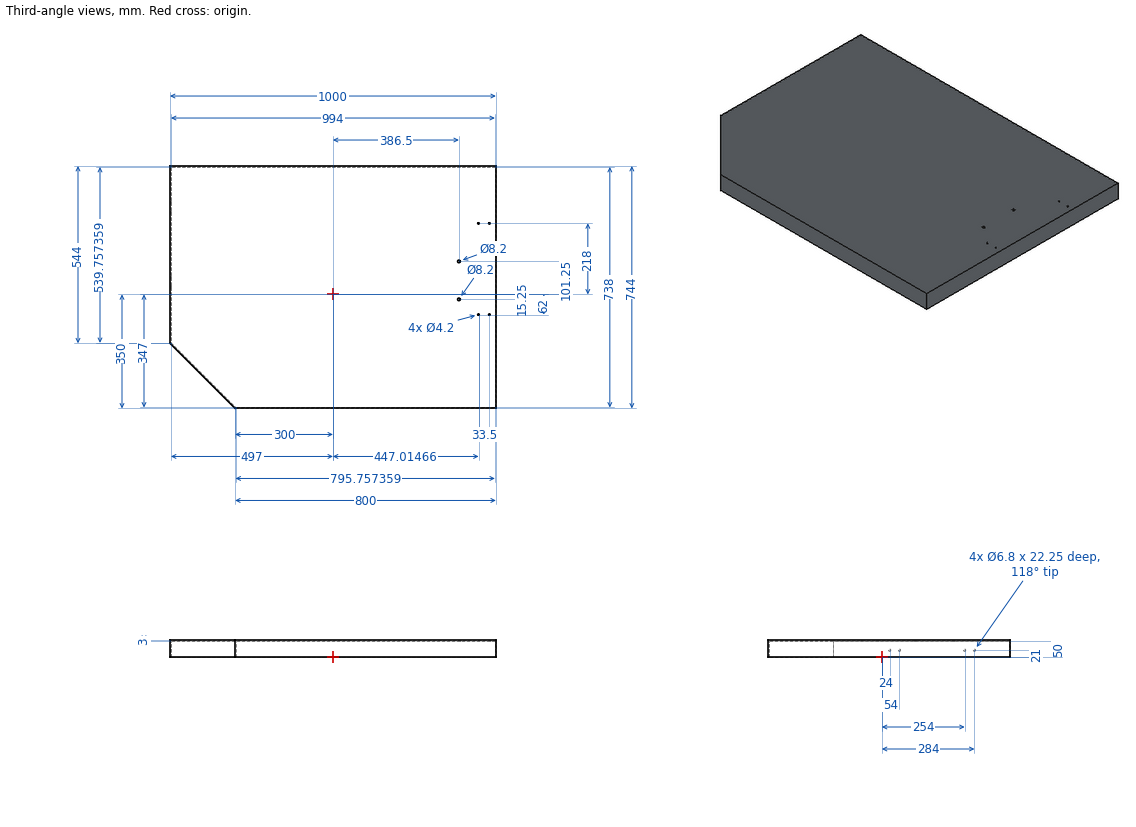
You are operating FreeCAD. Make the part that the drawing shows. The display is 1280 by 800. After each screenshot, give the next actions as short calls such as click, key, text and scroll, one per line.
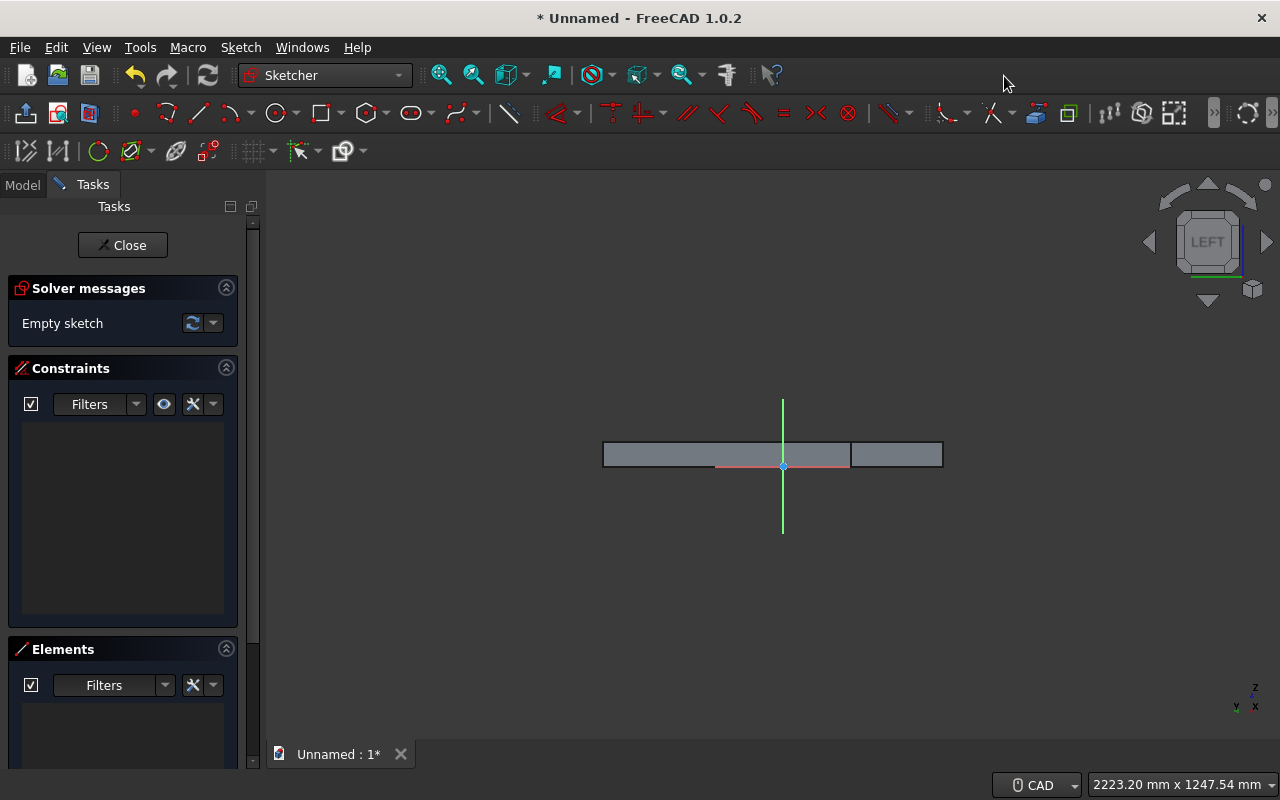
scroll(722, 463, up, 7)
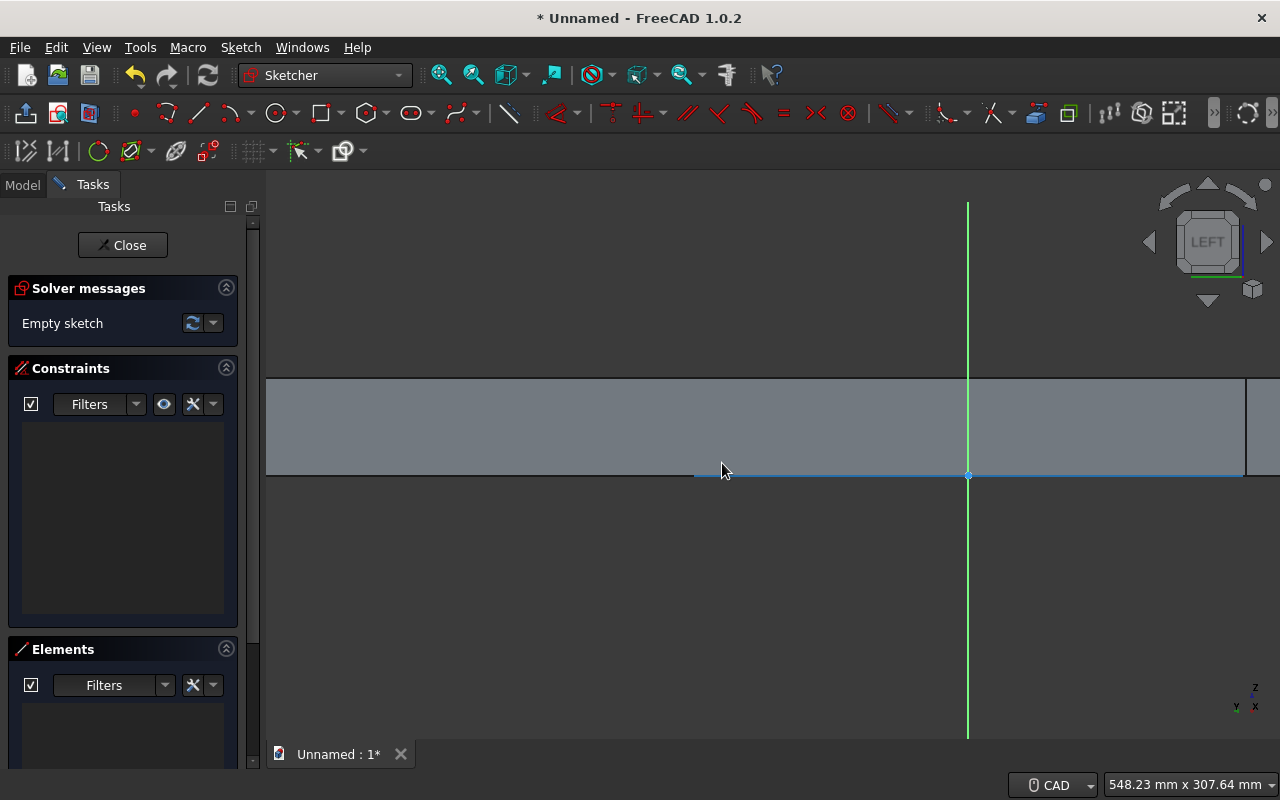
click(276, 114)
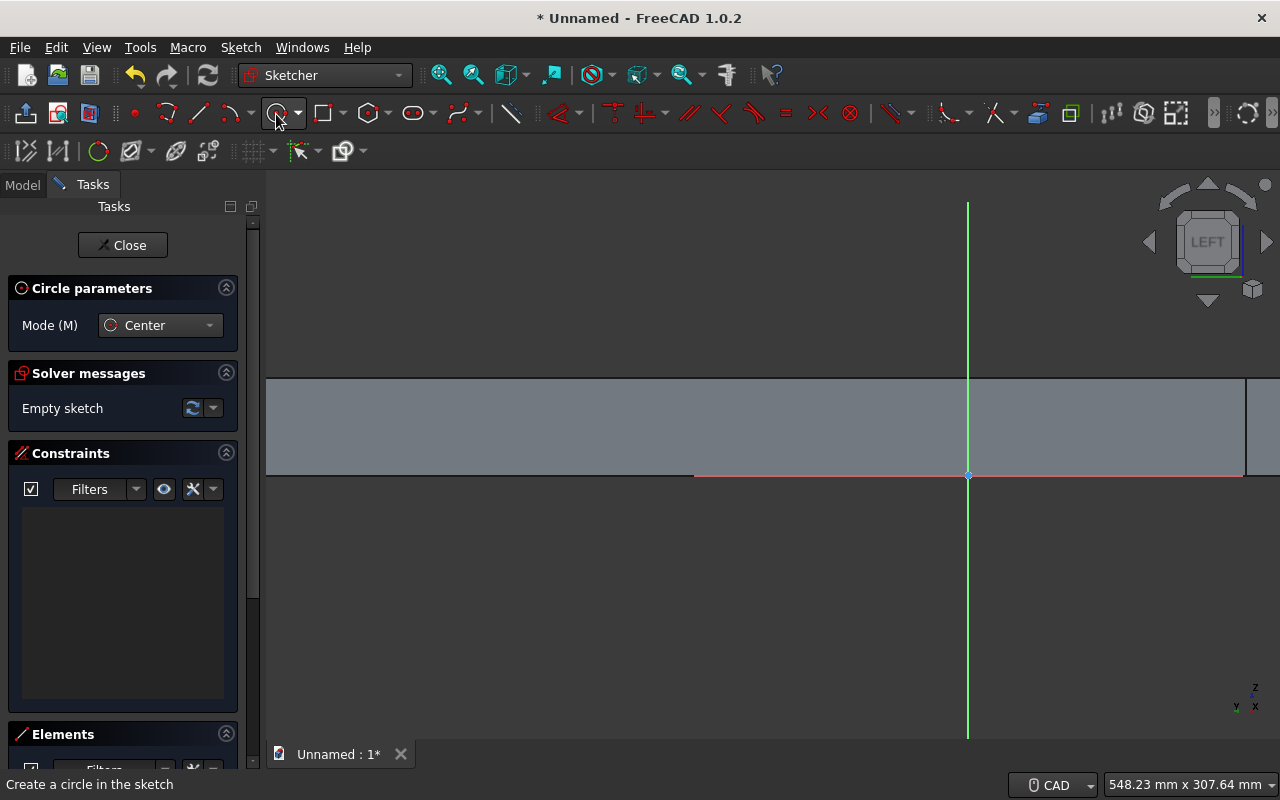
scroll(443, 437, up, 7)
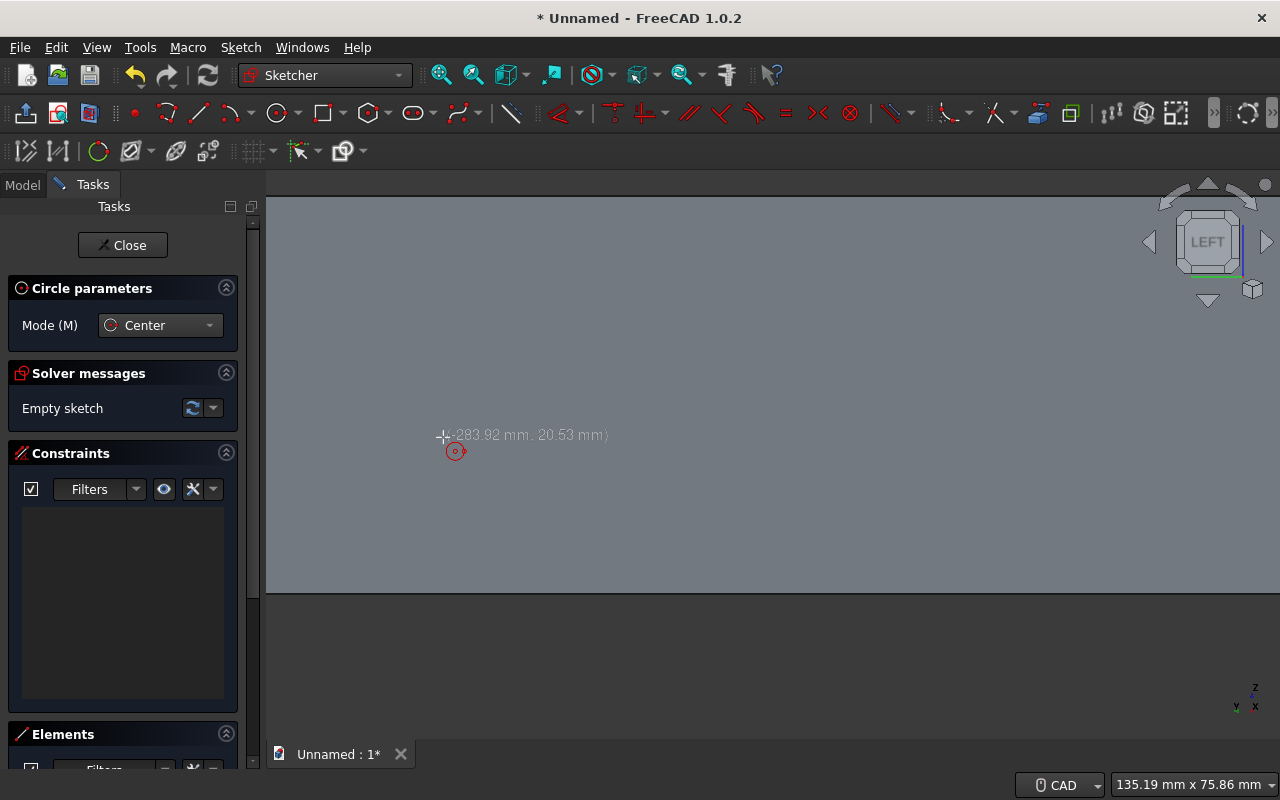
scroll(446, 439, down, 7)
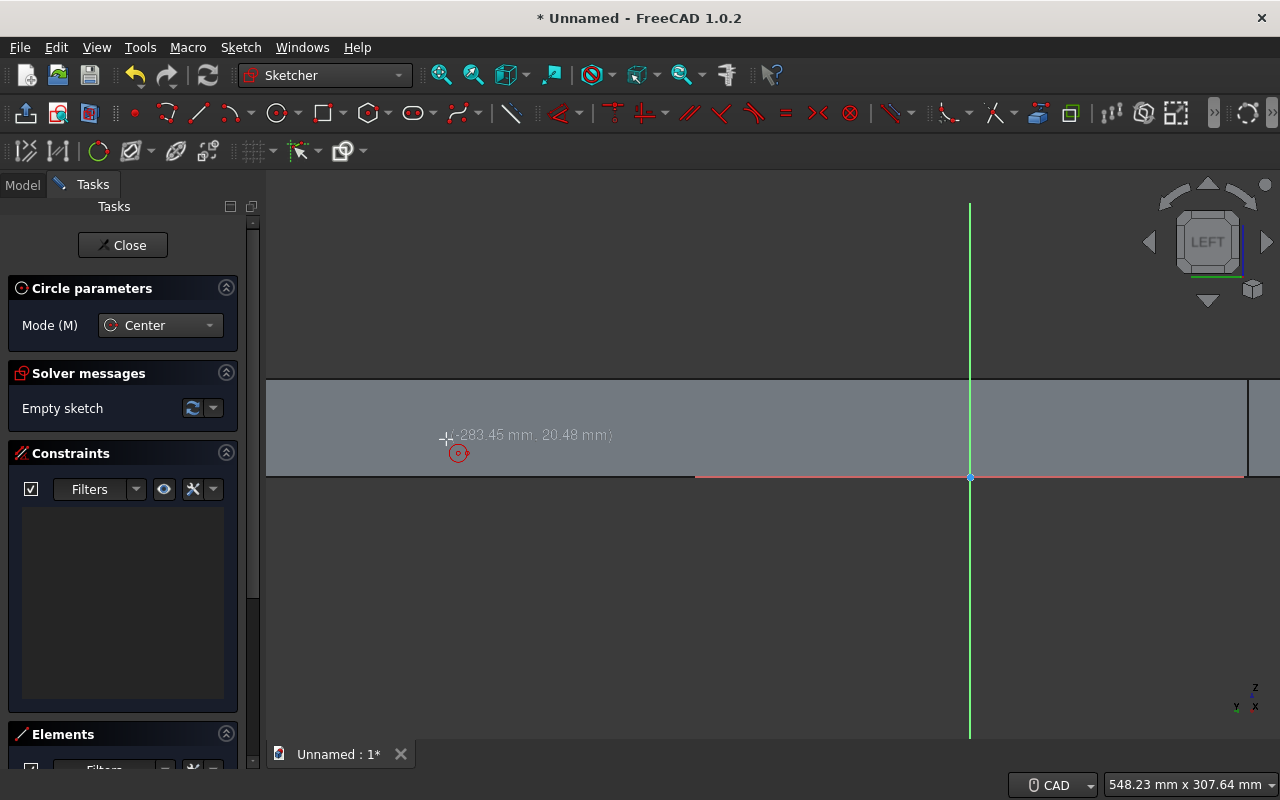
click(445, 439)
move(450, 434)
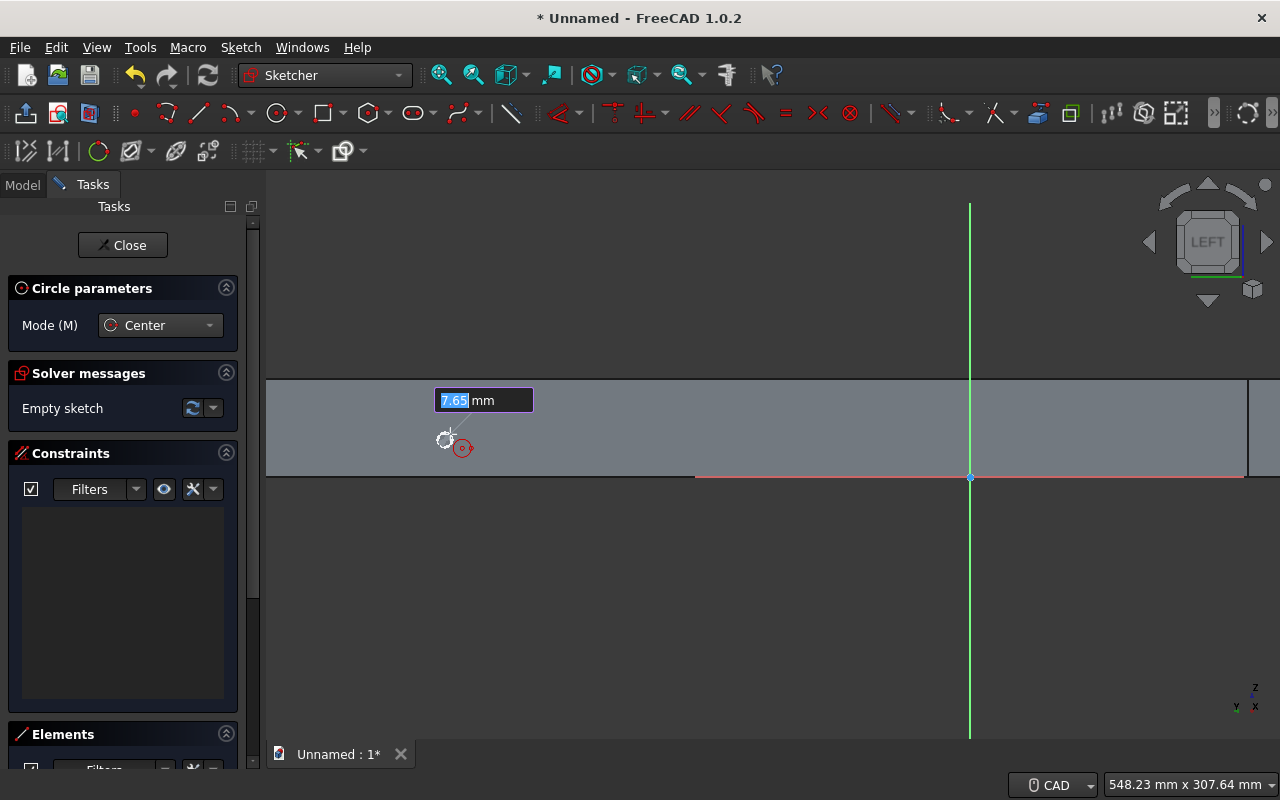
text(6.8)
key(Return)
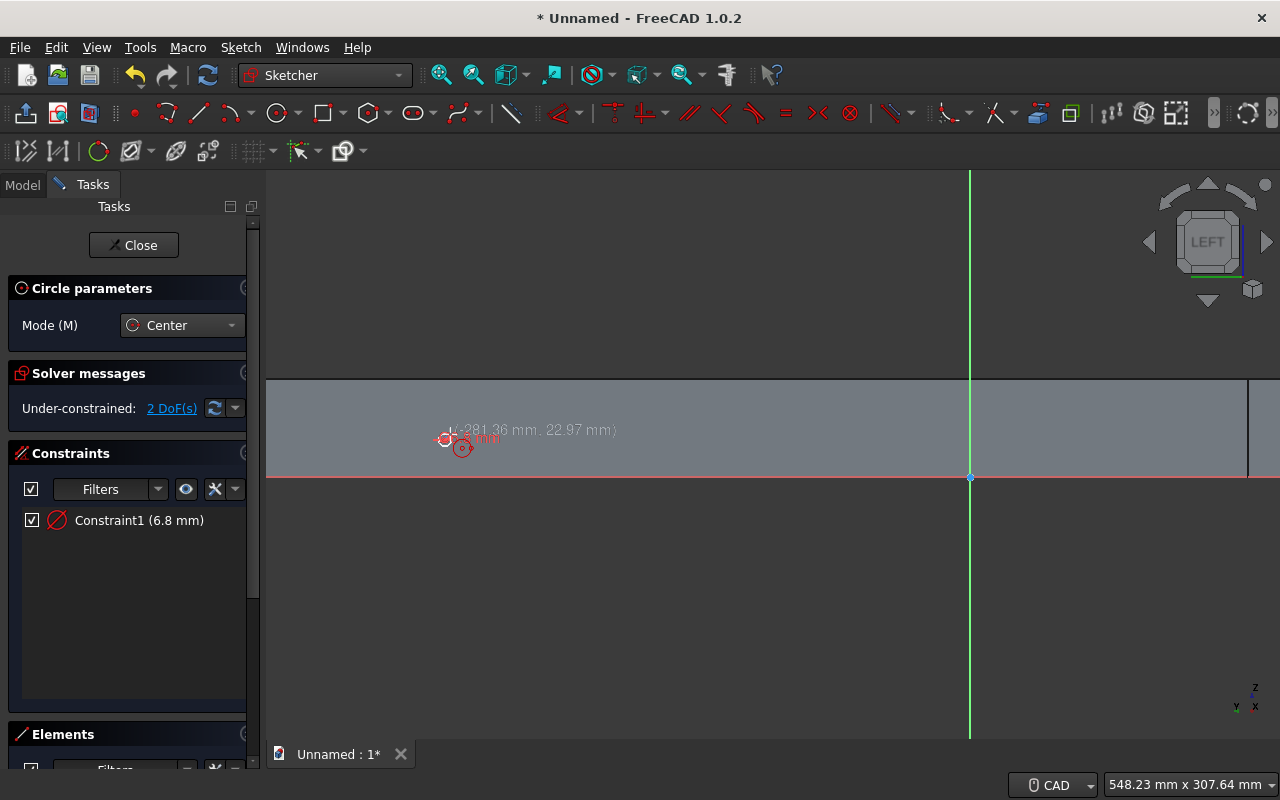
scroll(501, 439, up, 7)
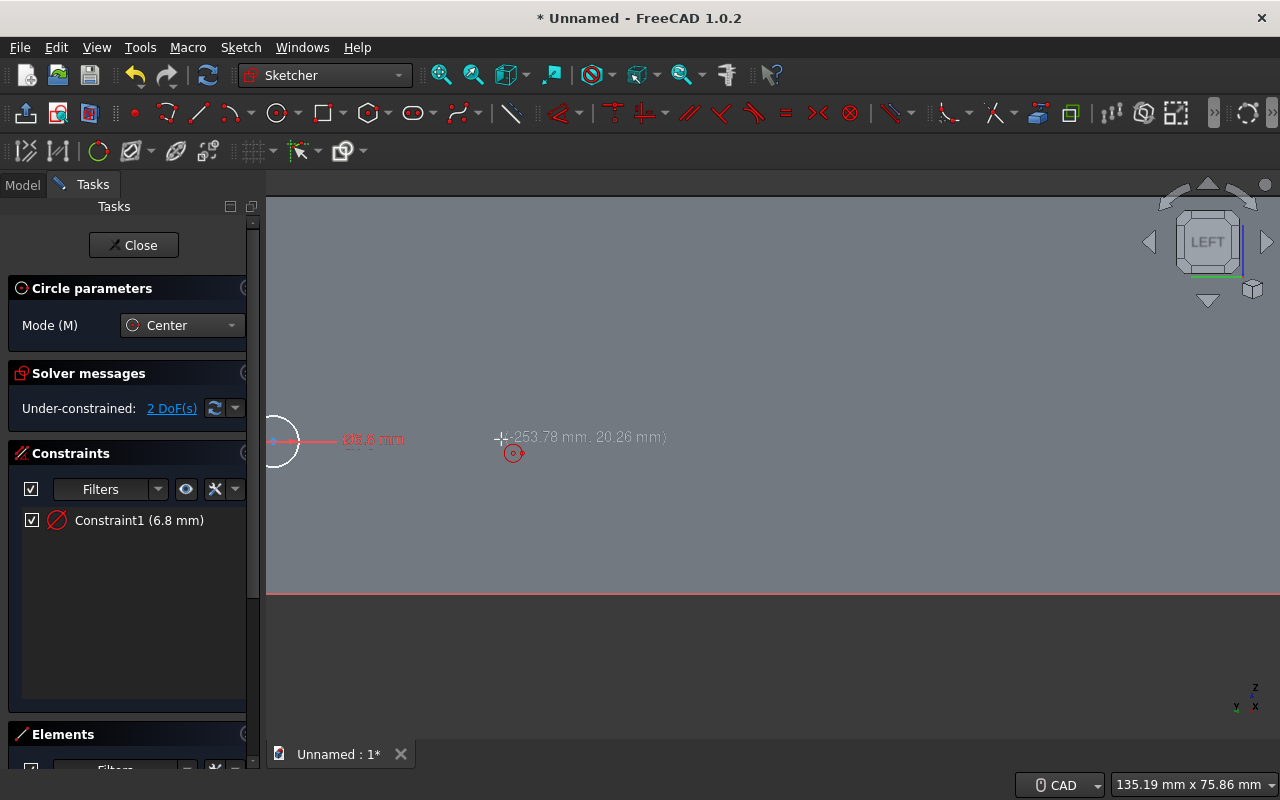
scroll(501, 439, down, 7)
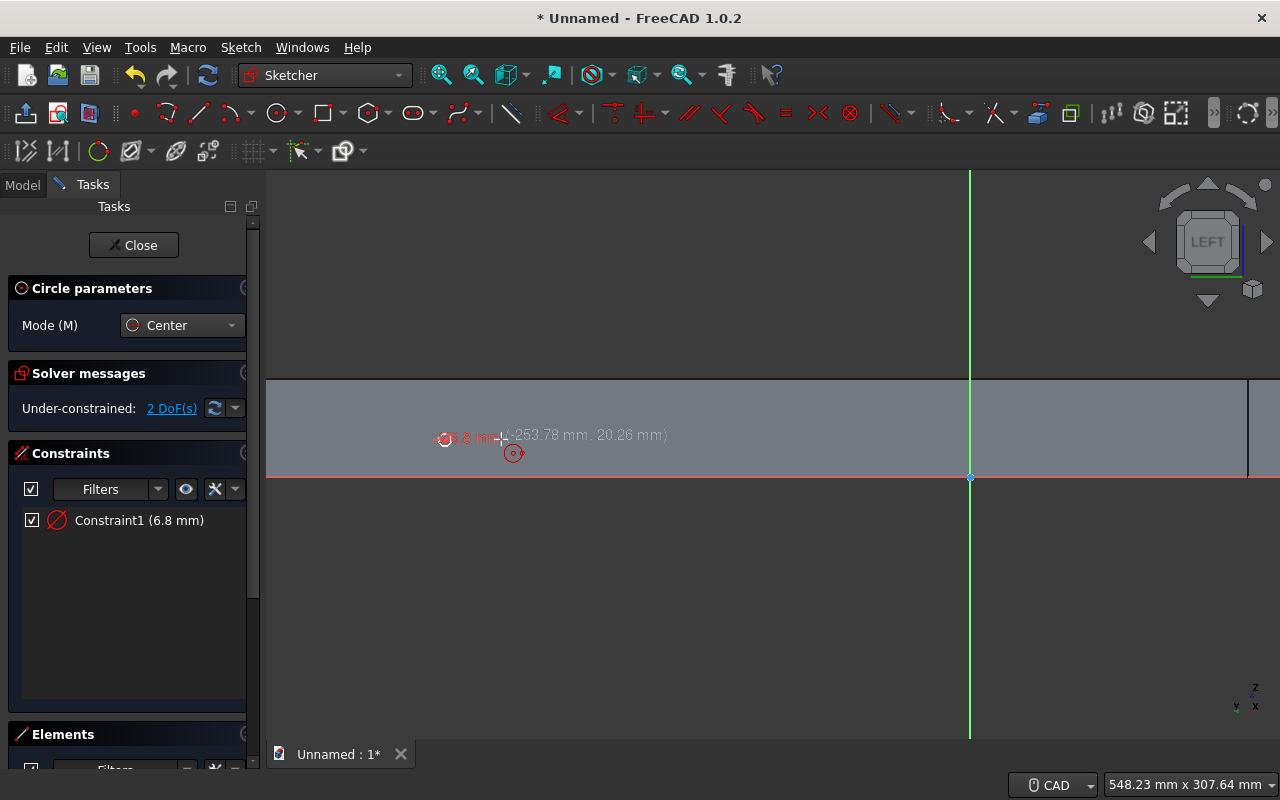
click(501, 439)
move(505, 434)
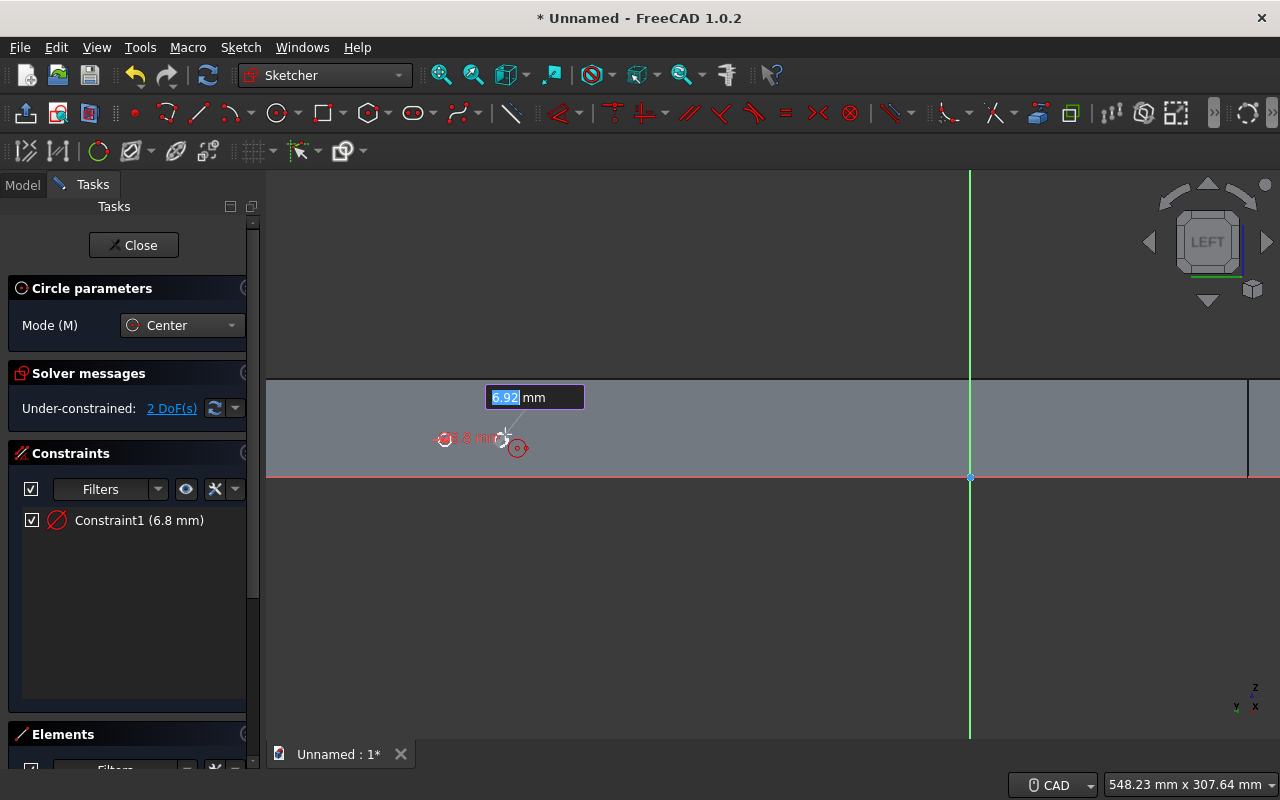
text(6.8)
key(Return)